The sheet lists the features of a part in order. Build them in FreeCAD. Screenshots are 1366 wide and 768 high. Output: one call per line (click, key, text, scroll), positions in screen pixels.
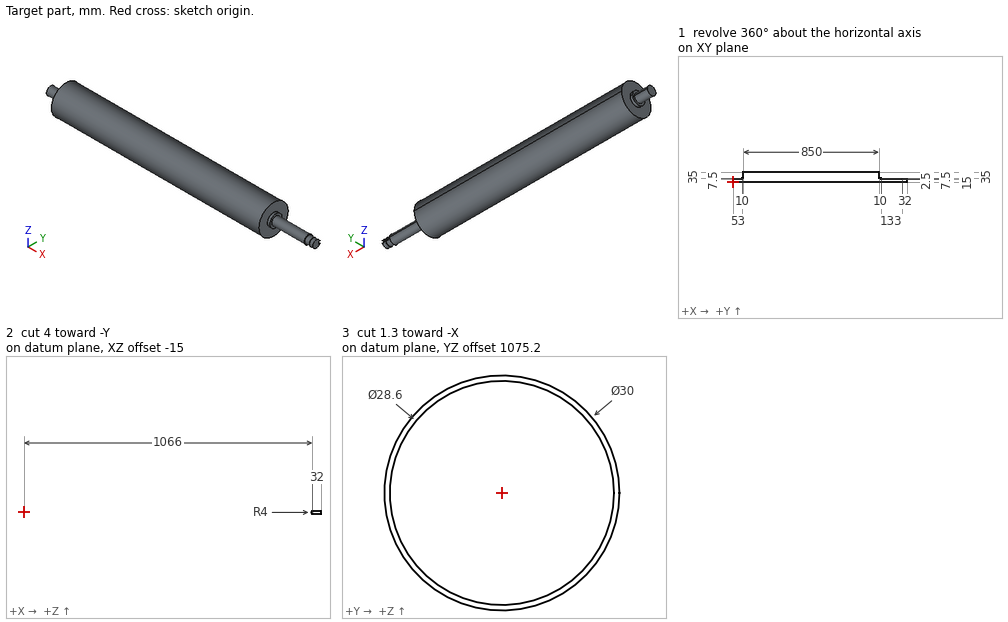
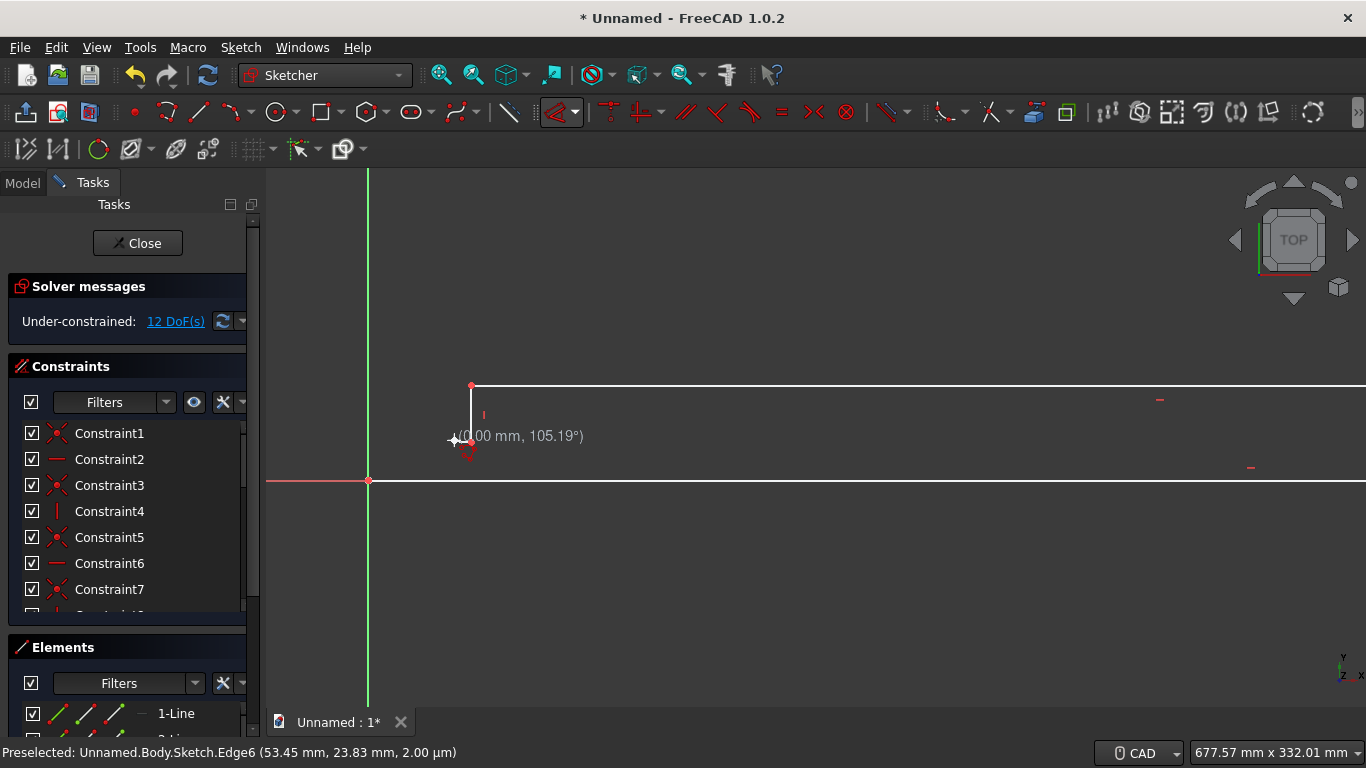
scroll(454, 452, up, 2)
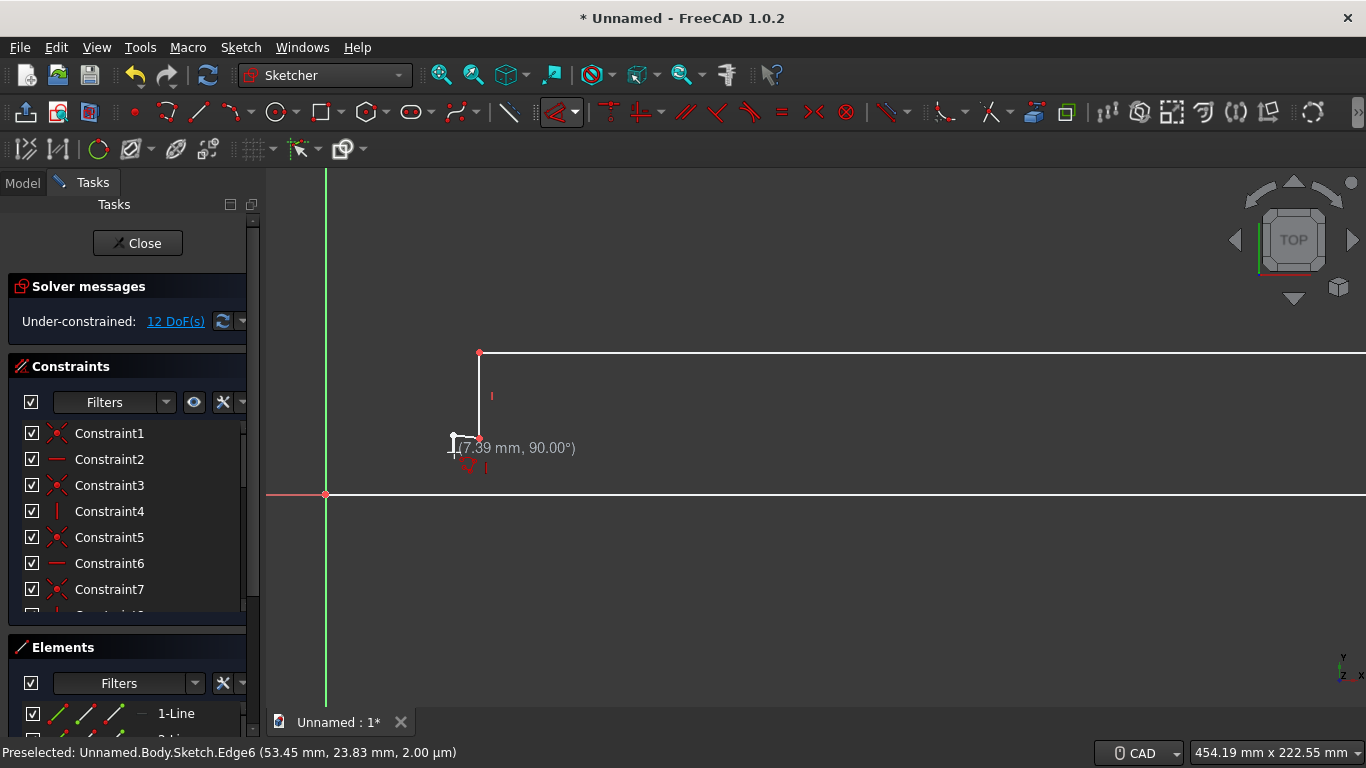
click(454, 452)
click(335, 452)
click(326, 495)
key(Escape)
key(Escape)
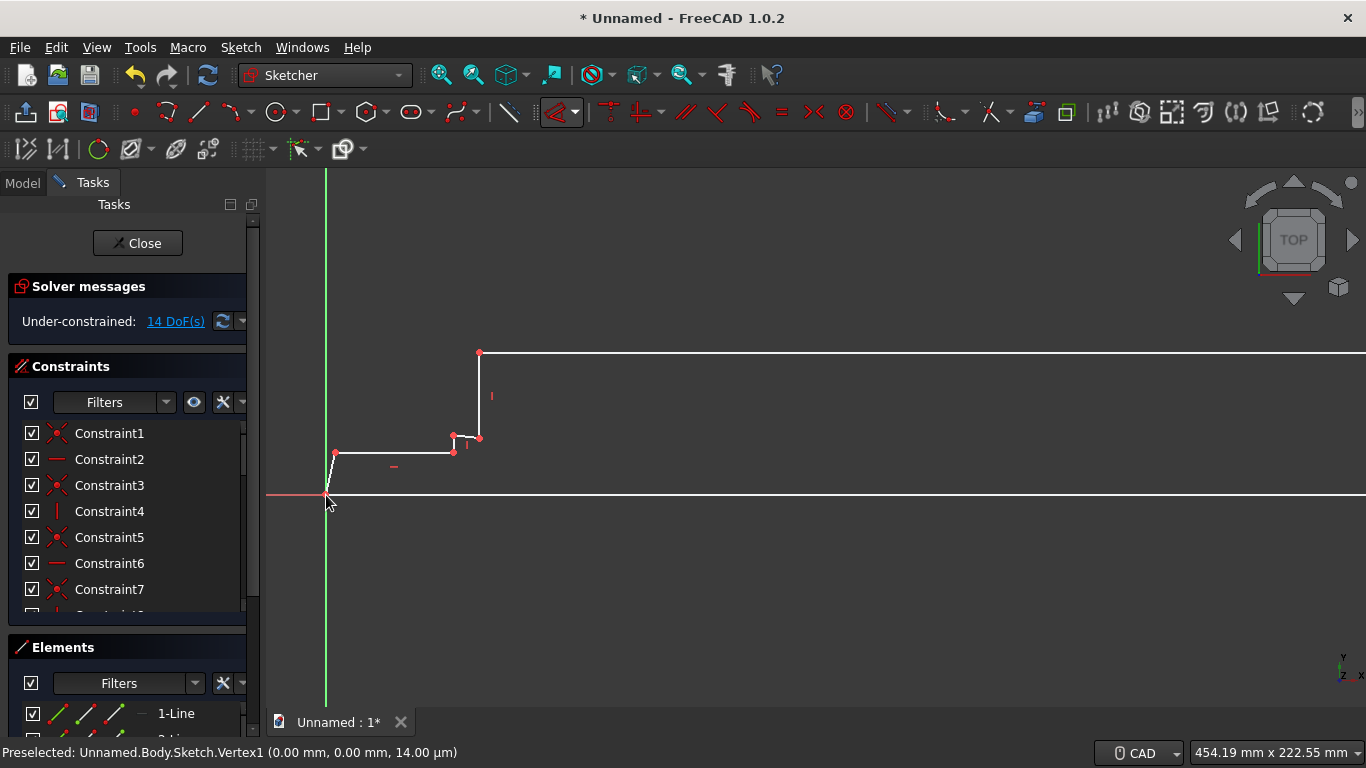
scroll(469, 437, up, 2)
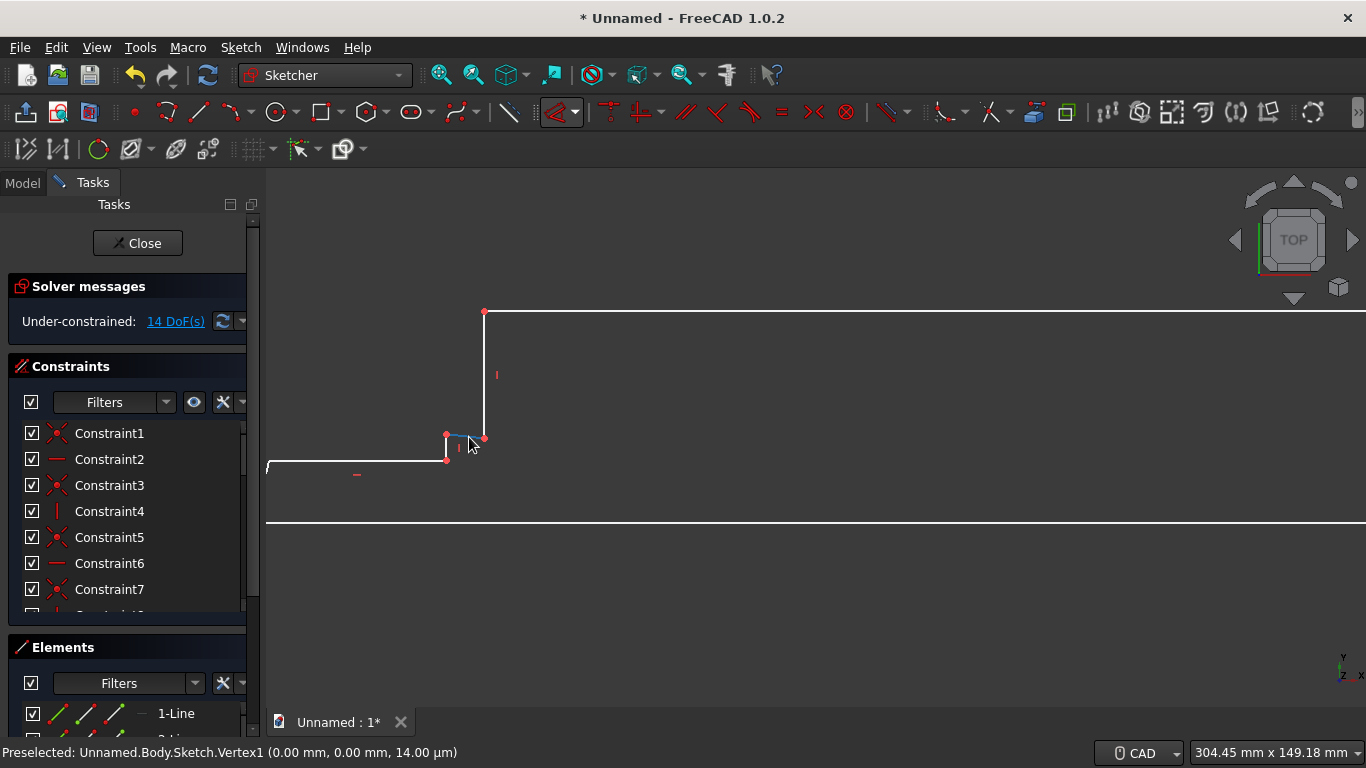
click(469, 437)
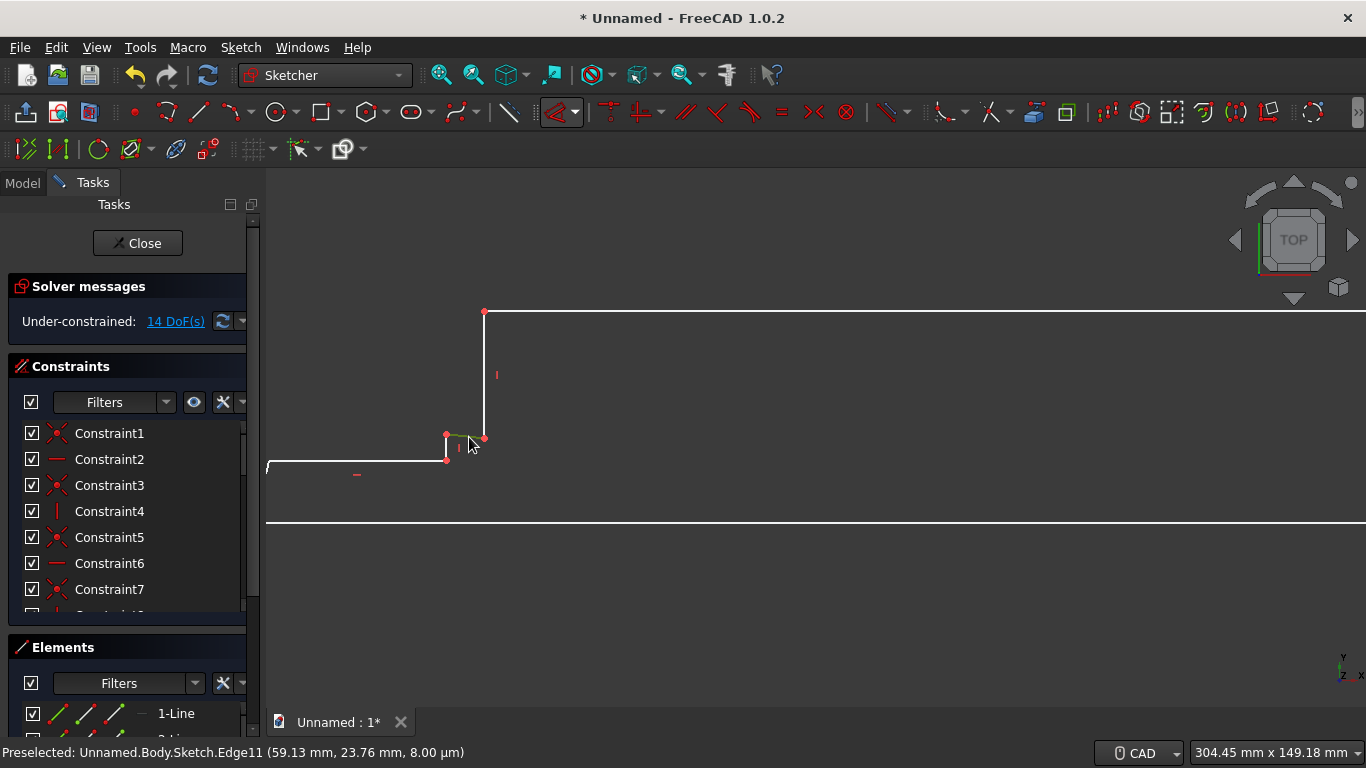
key(h)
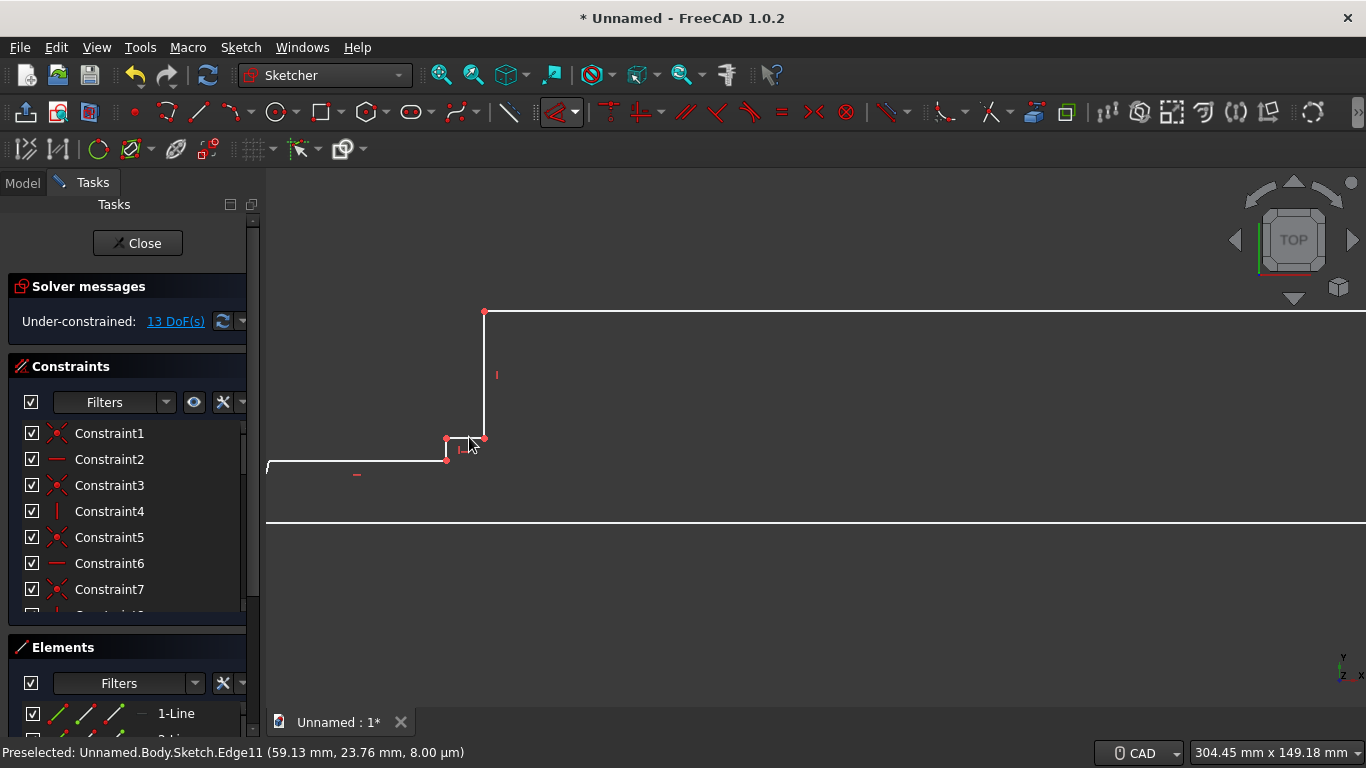
scroll(456, 442, down, 9)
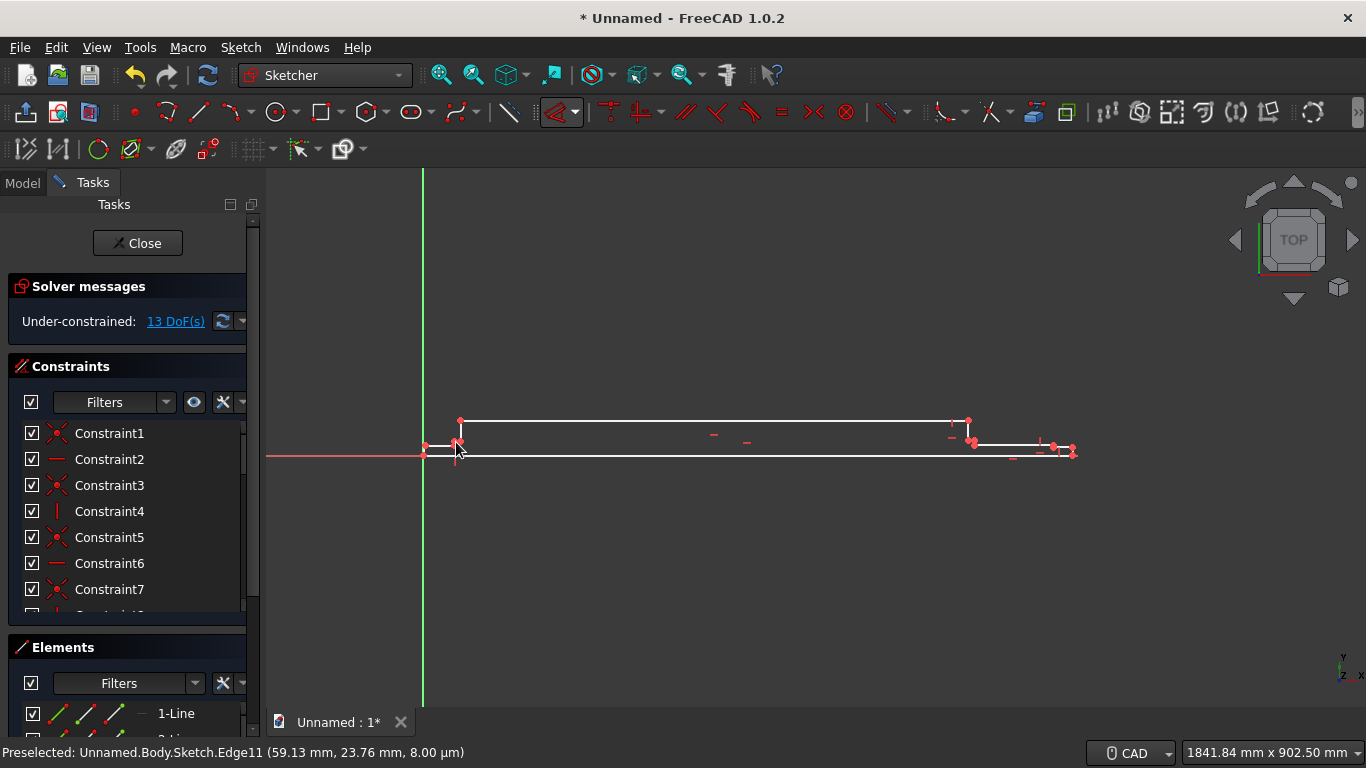
scroll(425, 449, up, 11)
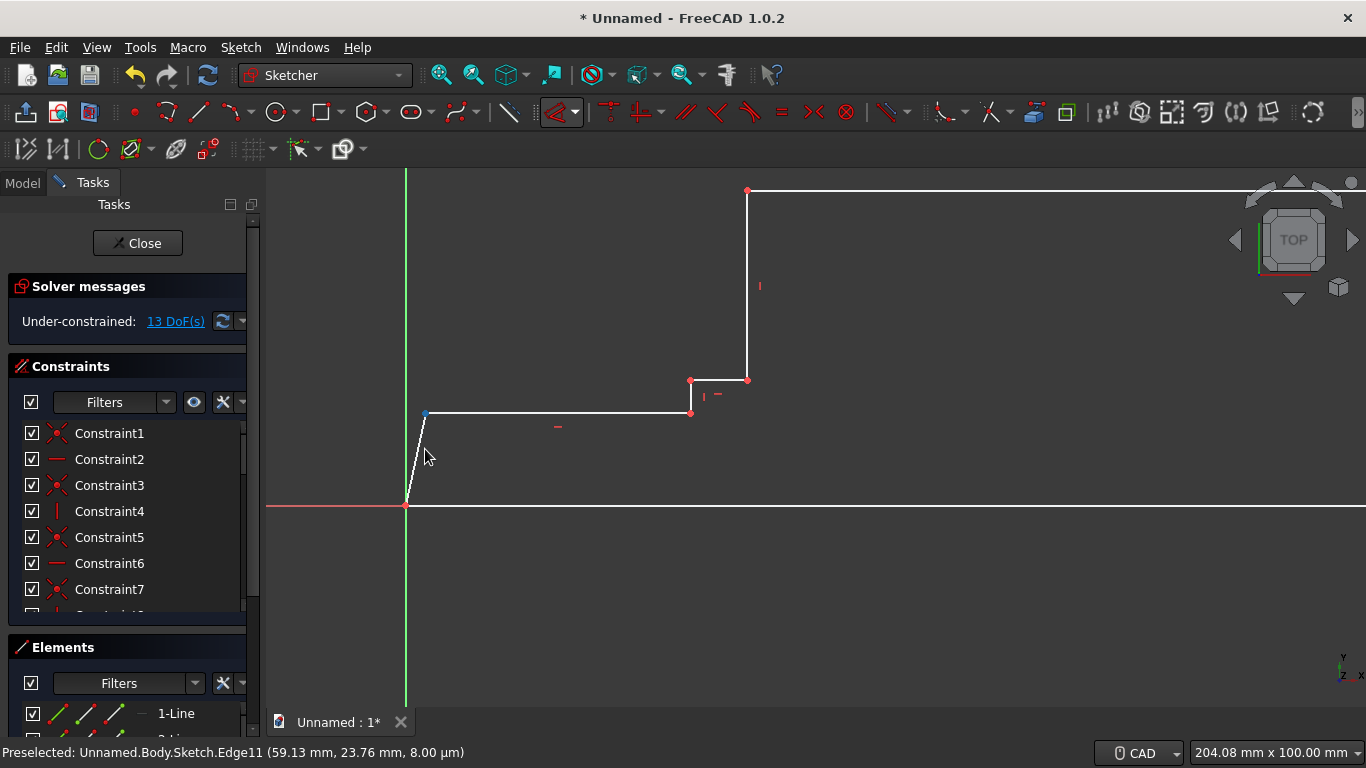
click(420, 441)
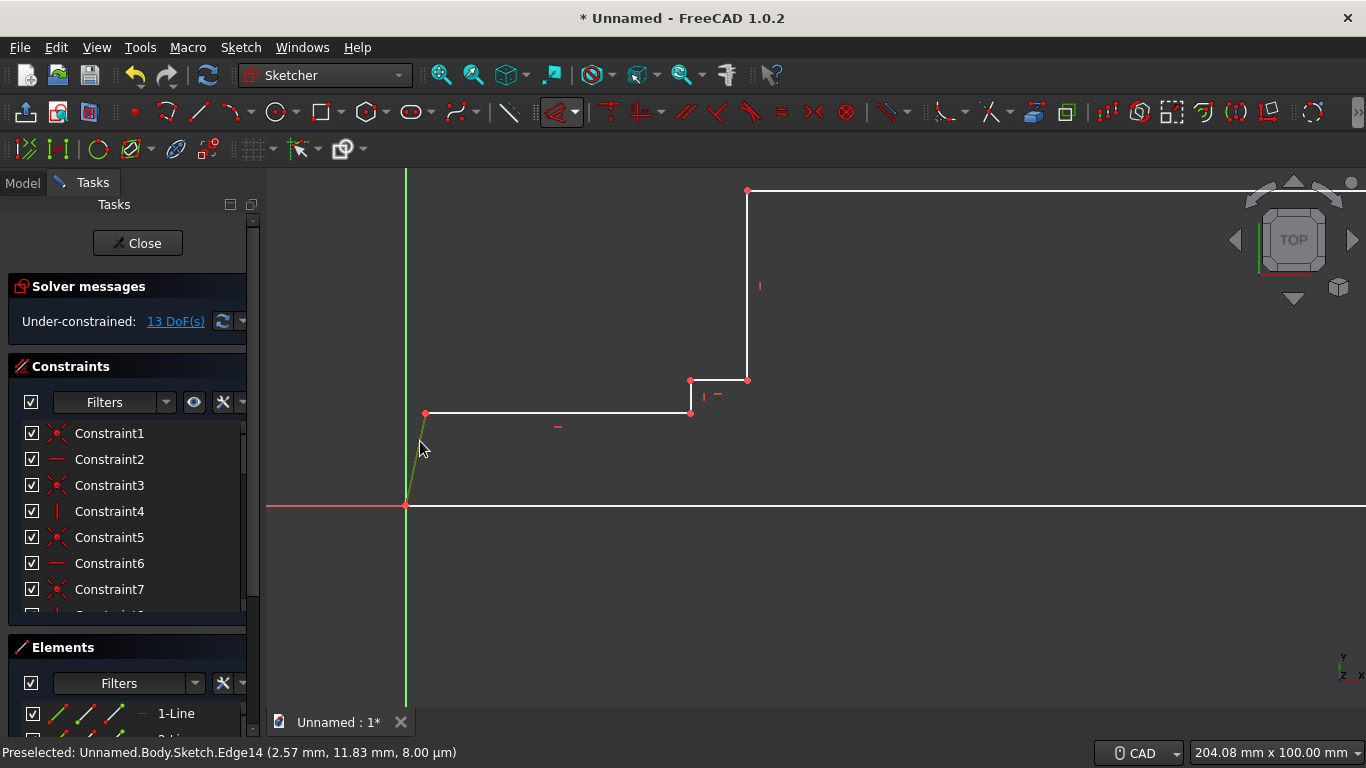
click(664, 112)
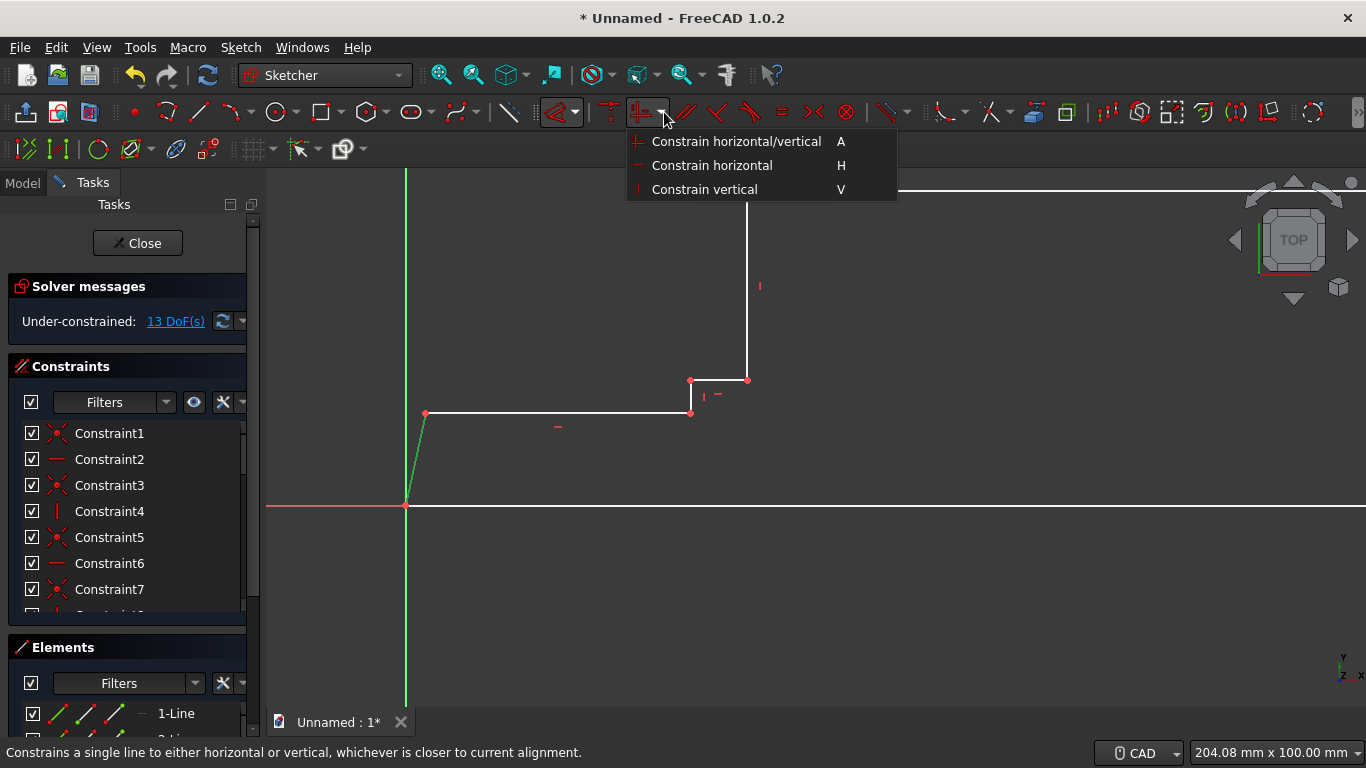
click(762, 189)